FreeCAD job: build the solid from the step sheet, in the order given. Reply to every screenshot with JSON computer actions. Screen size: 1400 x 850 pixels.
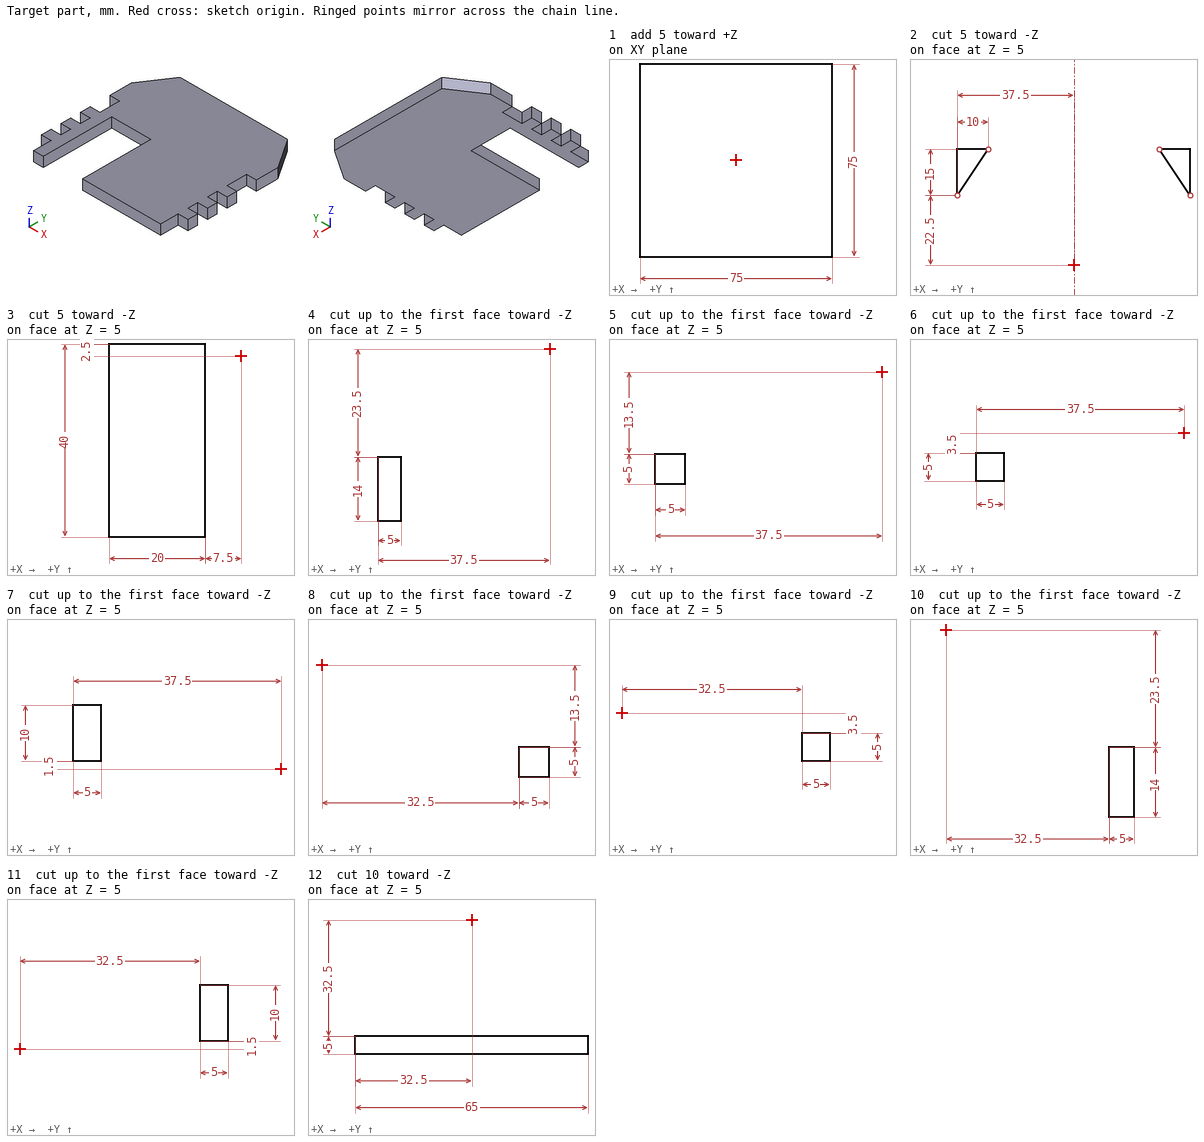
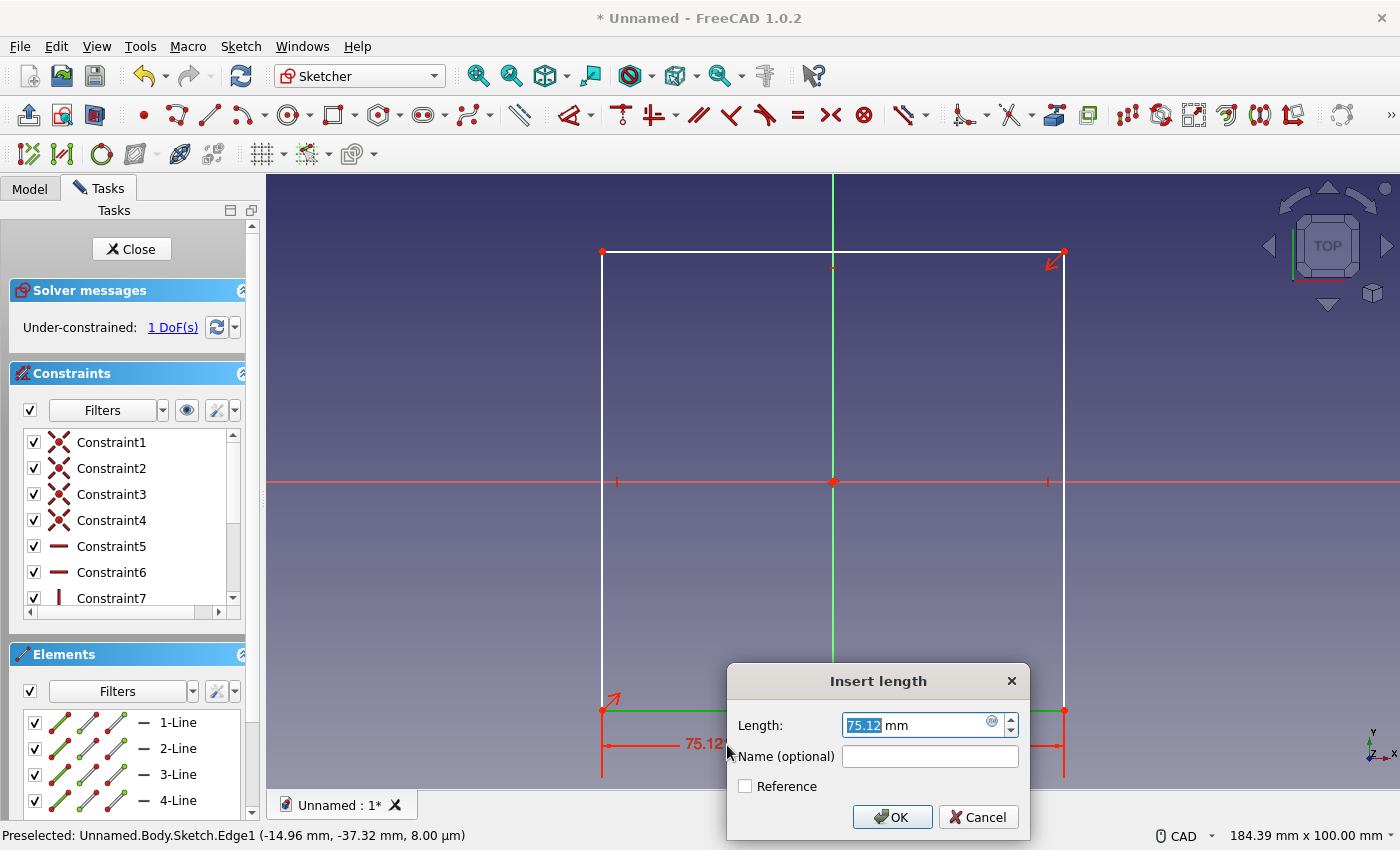
{"action": "type", "text": "75"}
{"action": "key", "text": "Return"}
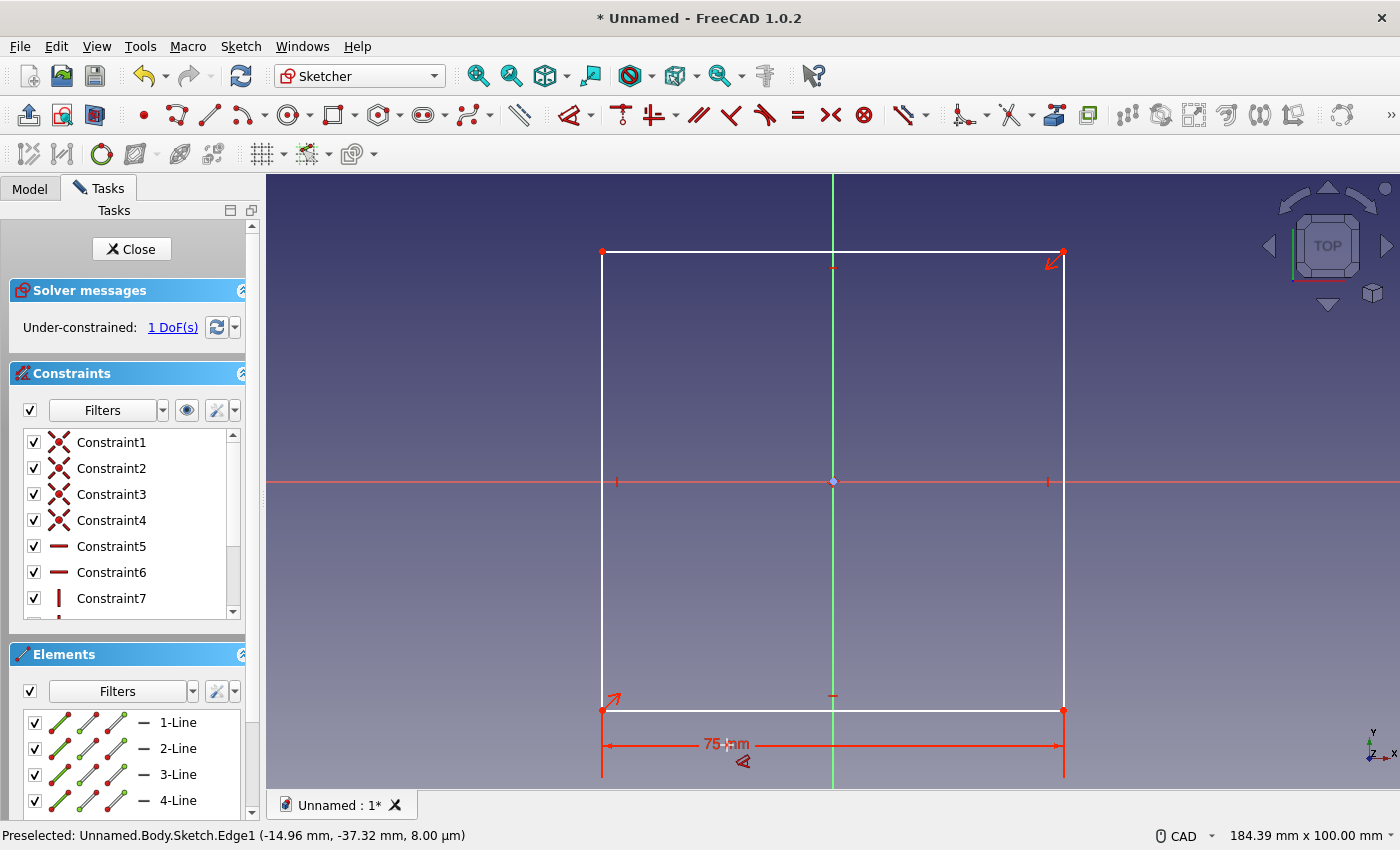
{"action": "left_click", "coordinate": [1064, 573]}
{"action": "left_click", "coordinate": [1098, 376]}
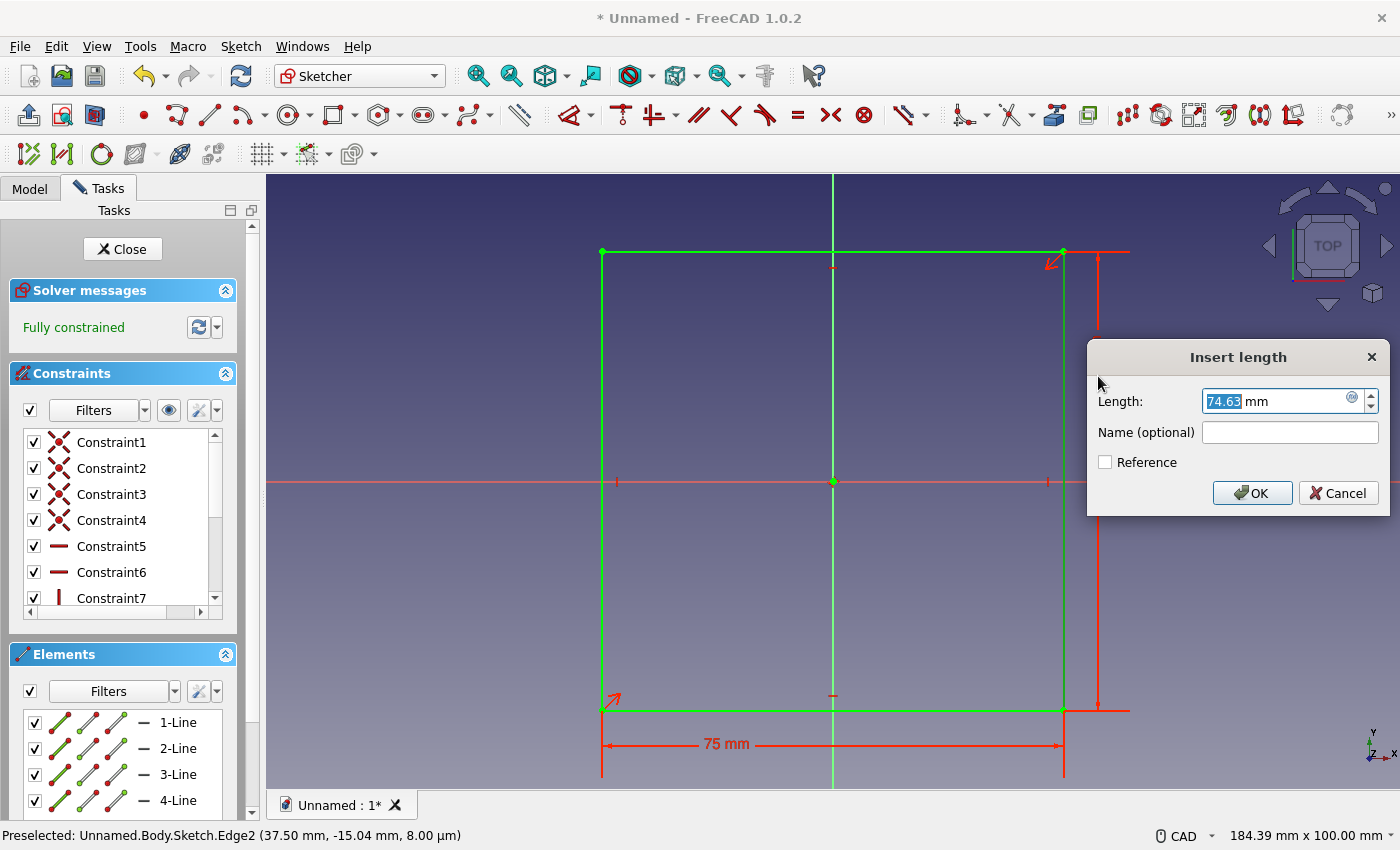
{"action": "type", "text": "75"}
{"action": "key", "text": "Return"}
{"action": "key", "text": "Escape"}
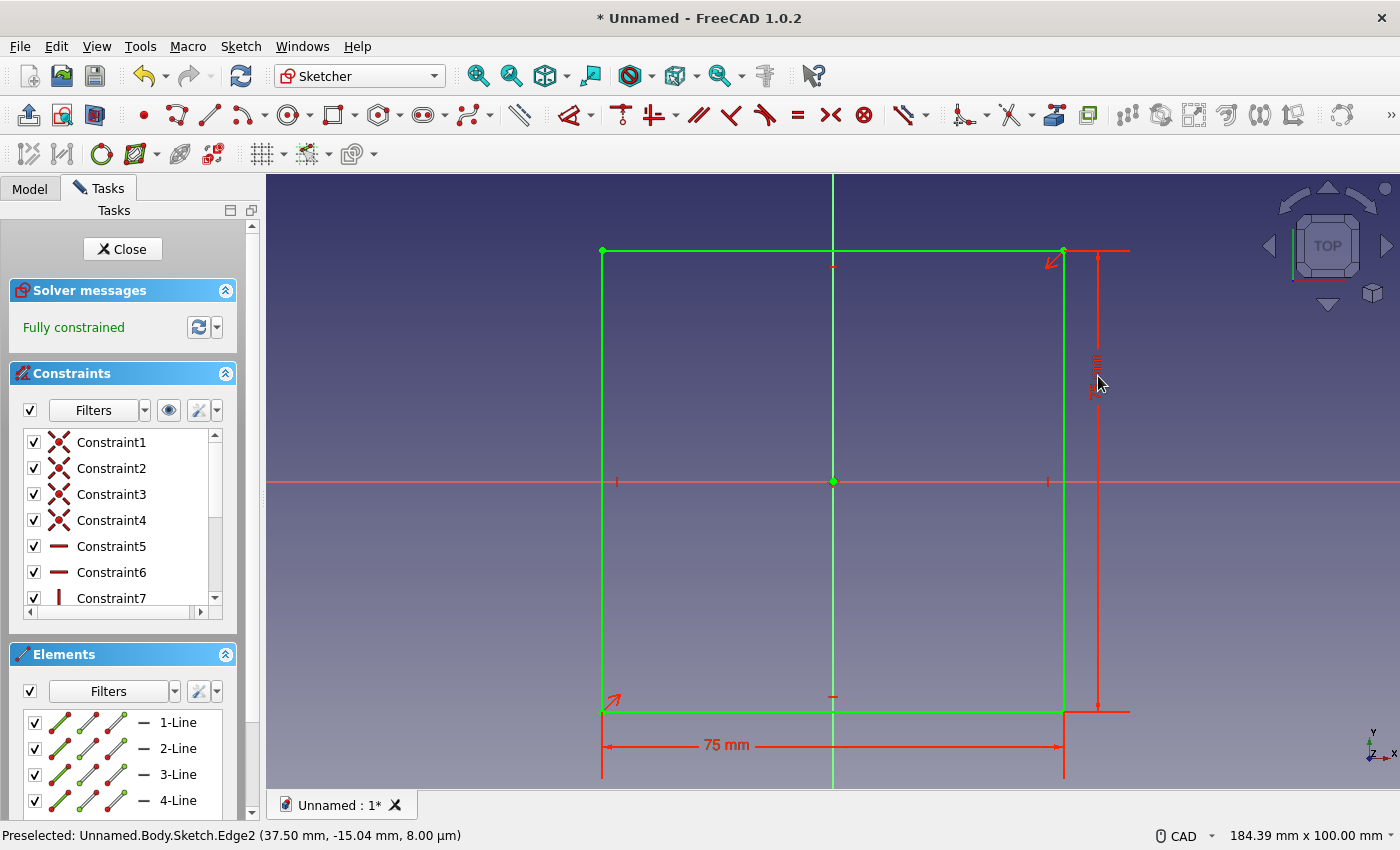
{"action": "left_click", "coordinate": [123, 249]}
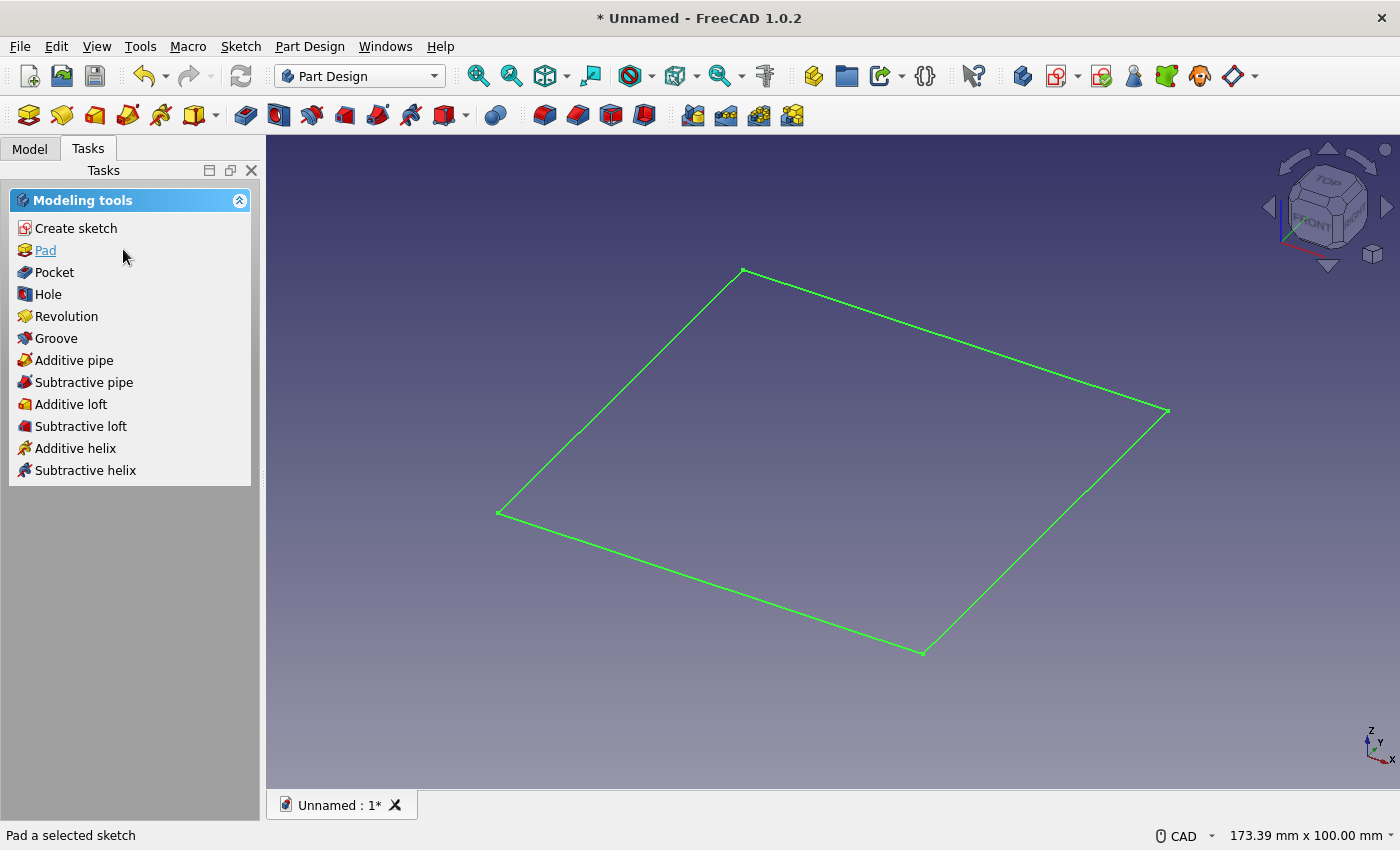
{"action": "left_click", "coordinate": [29, 116]}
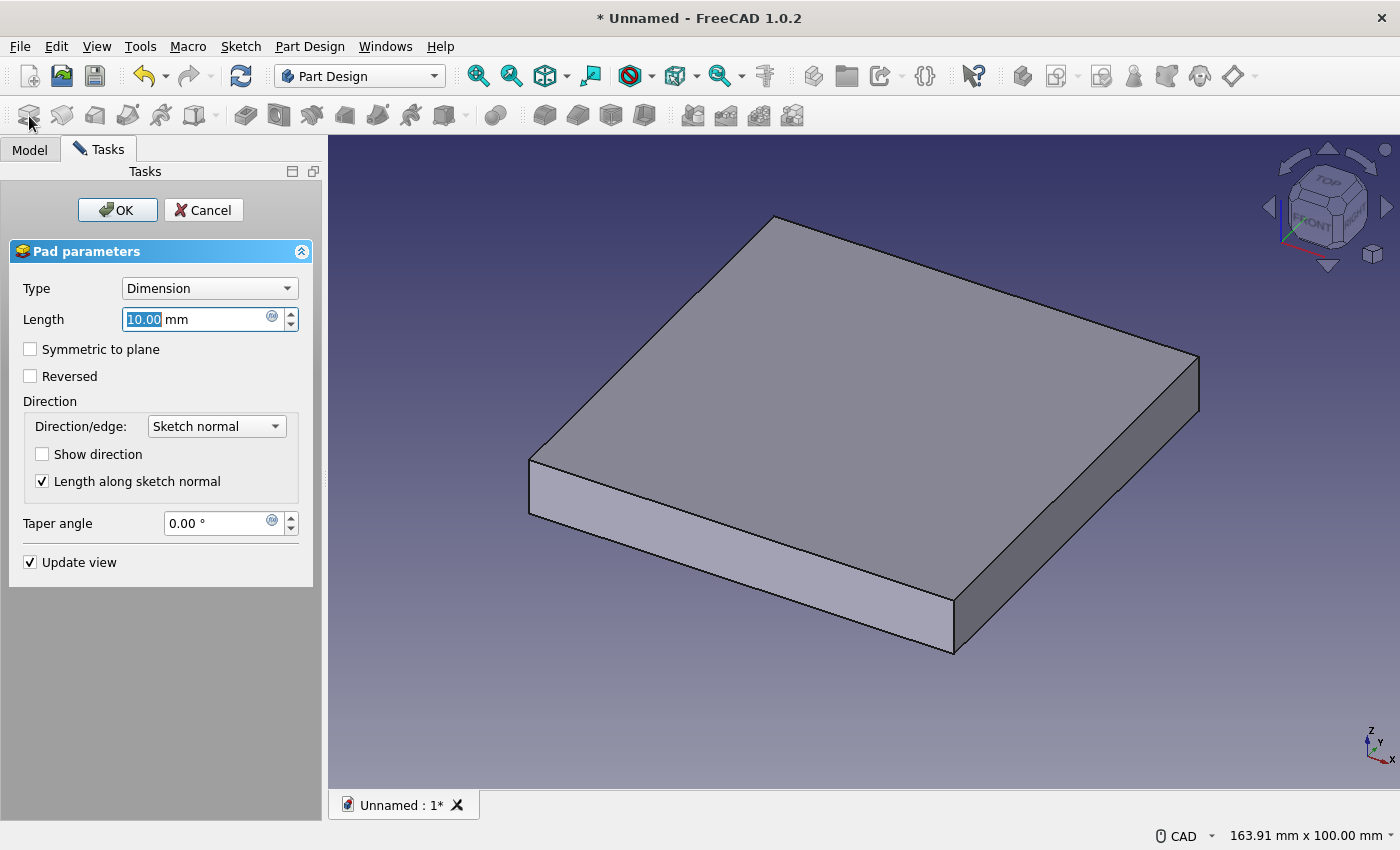
{"action": "type", "text": "5"}
{"action": "key", "text": "Tab"}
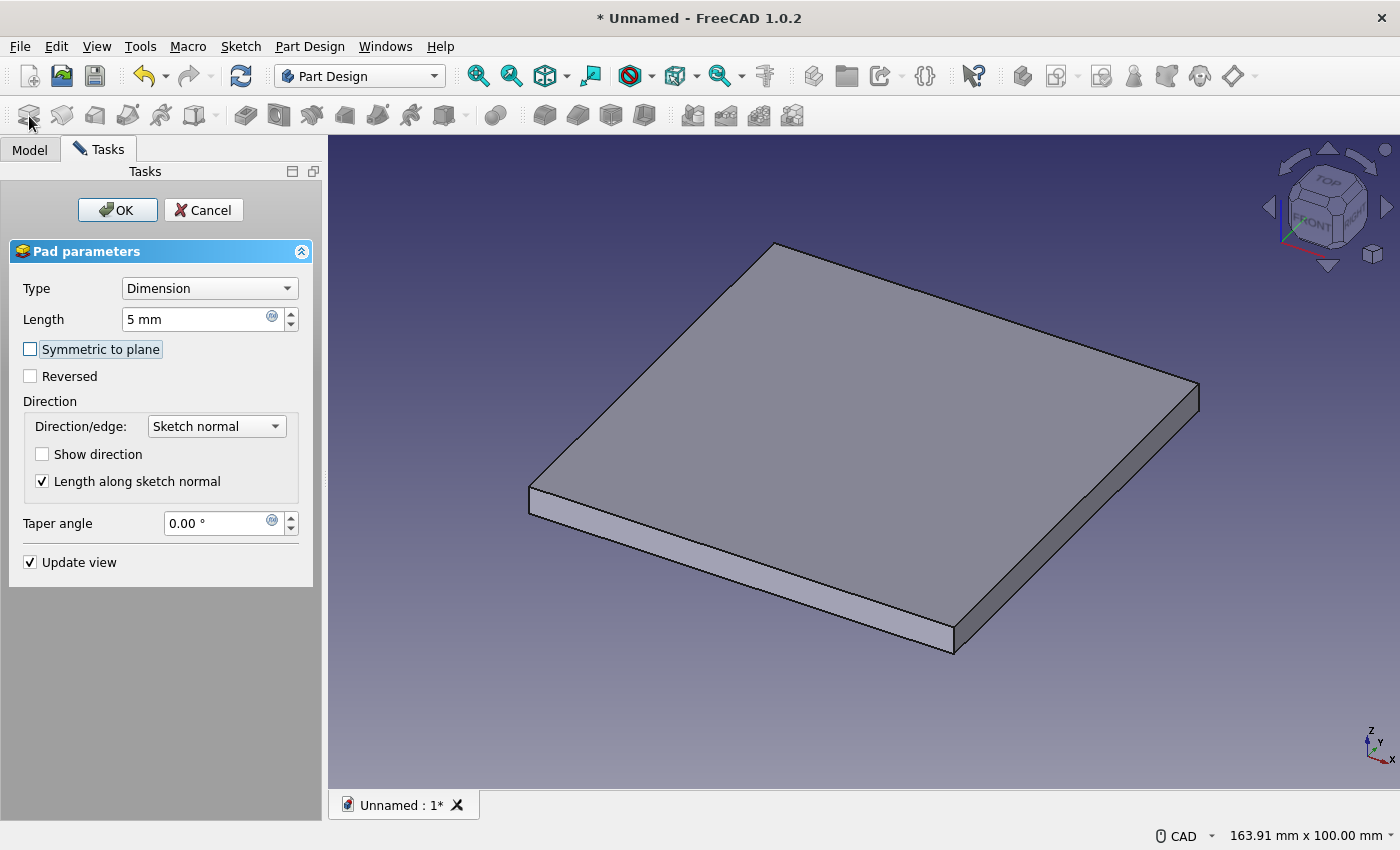
{"action": "left_click", "coordinate": [118, 210]}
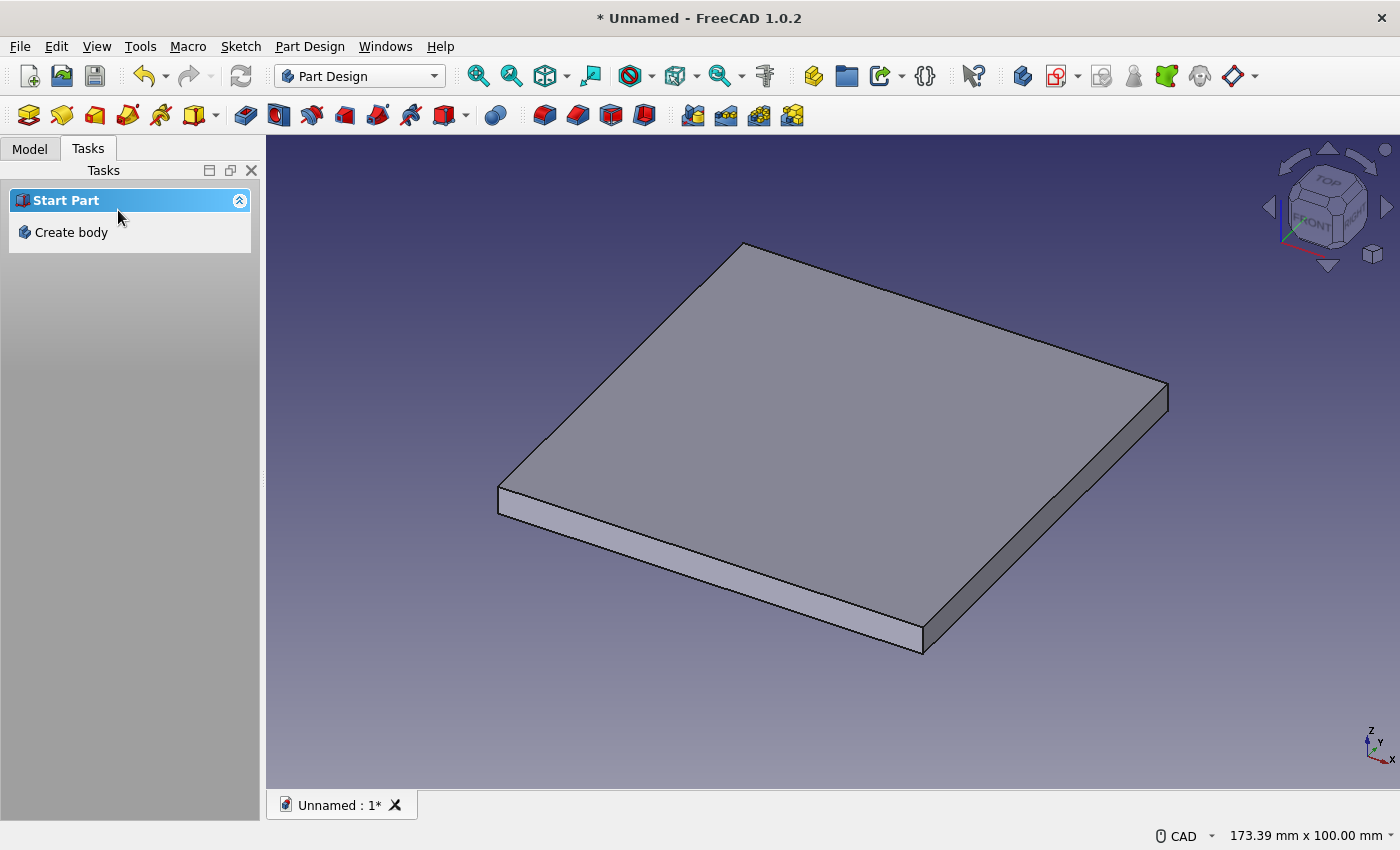
{"action": "left_click", "coordinate": [833, 434]}